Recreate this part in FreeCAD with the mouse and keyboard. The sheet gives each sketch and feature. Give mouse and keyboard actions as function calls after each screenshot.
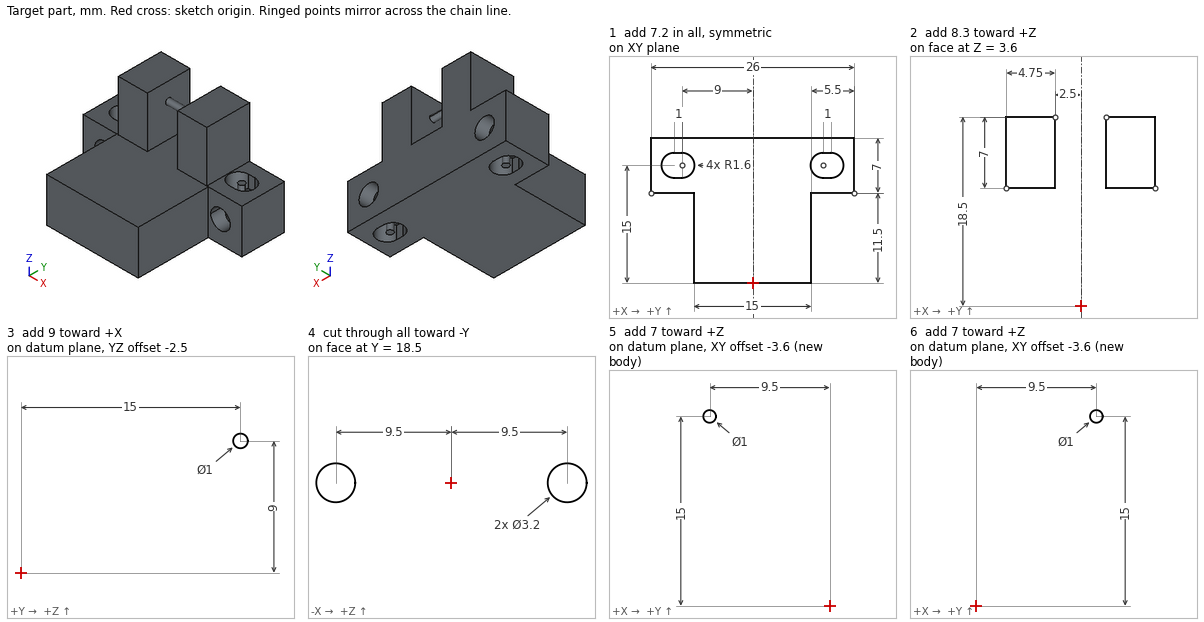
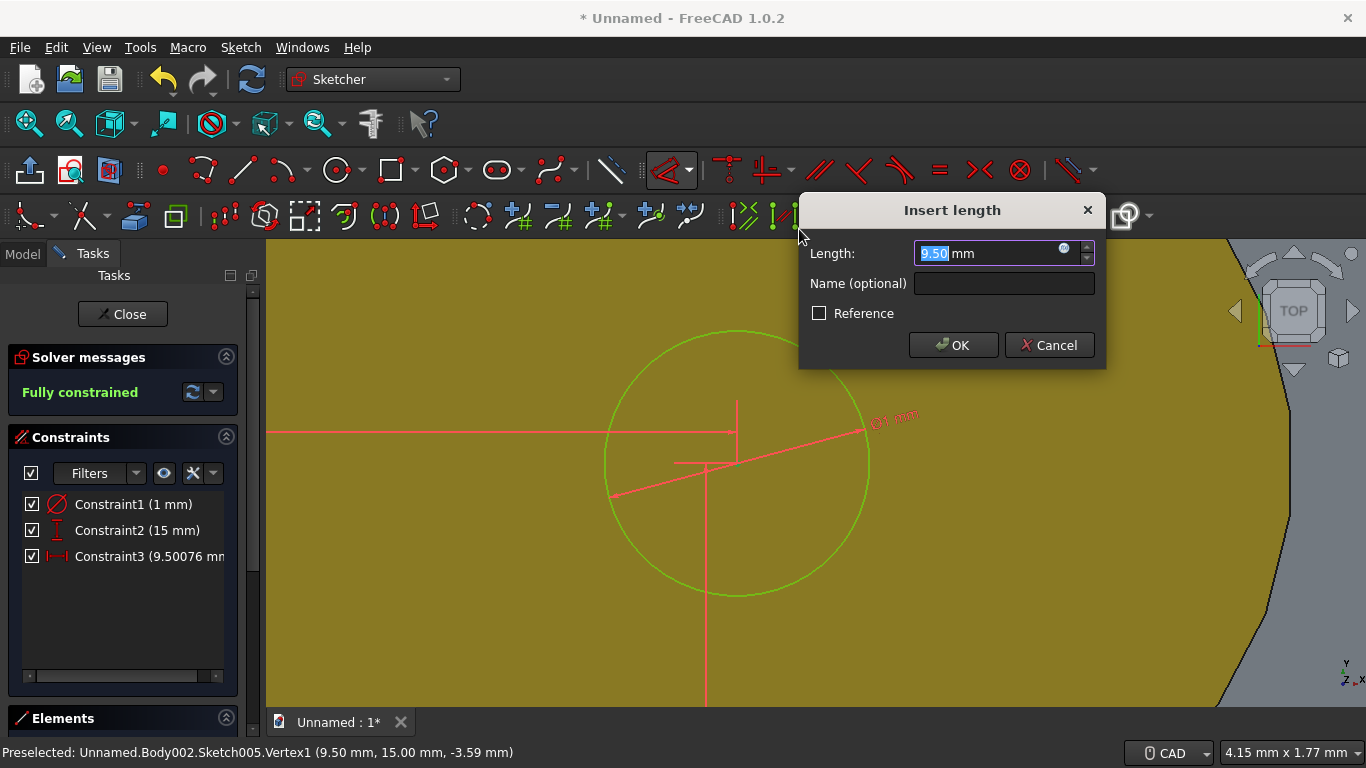
text(9.5)
key(Return)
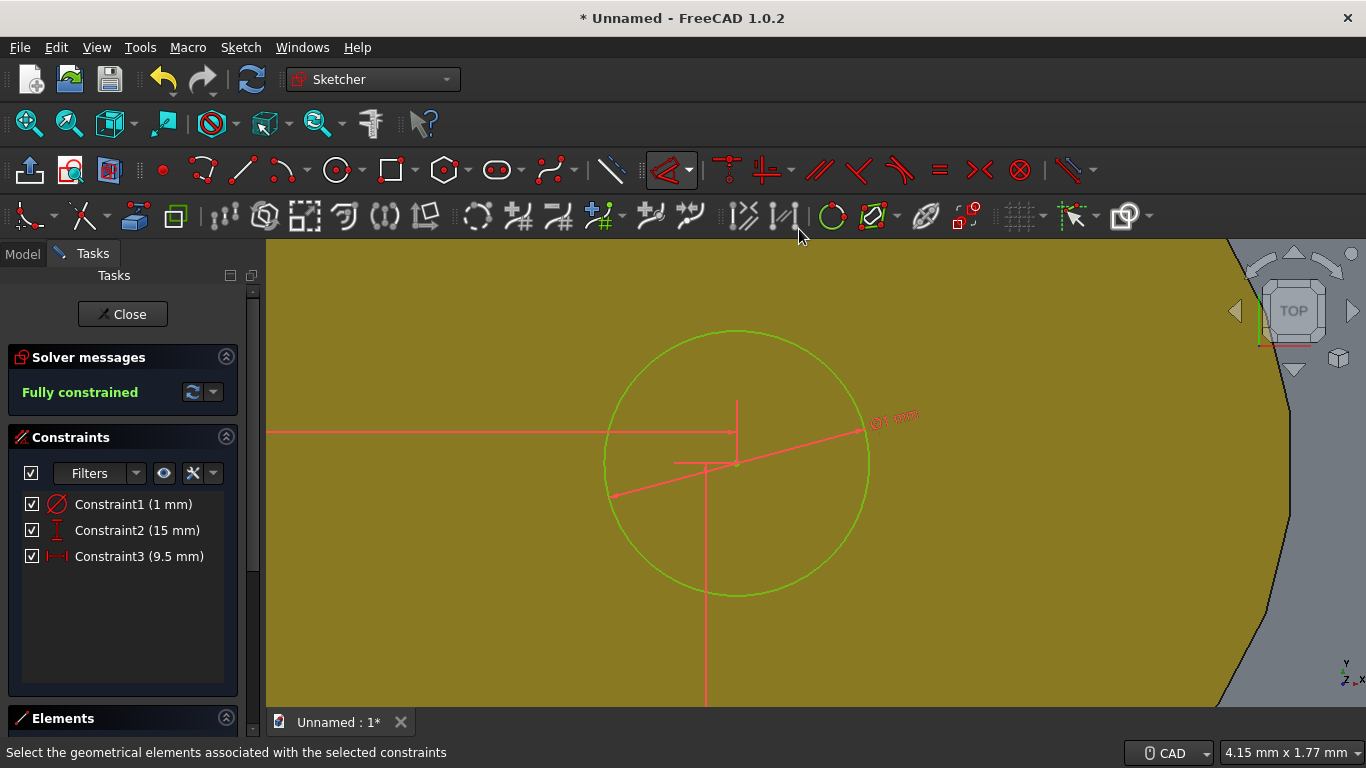
click(123, 314)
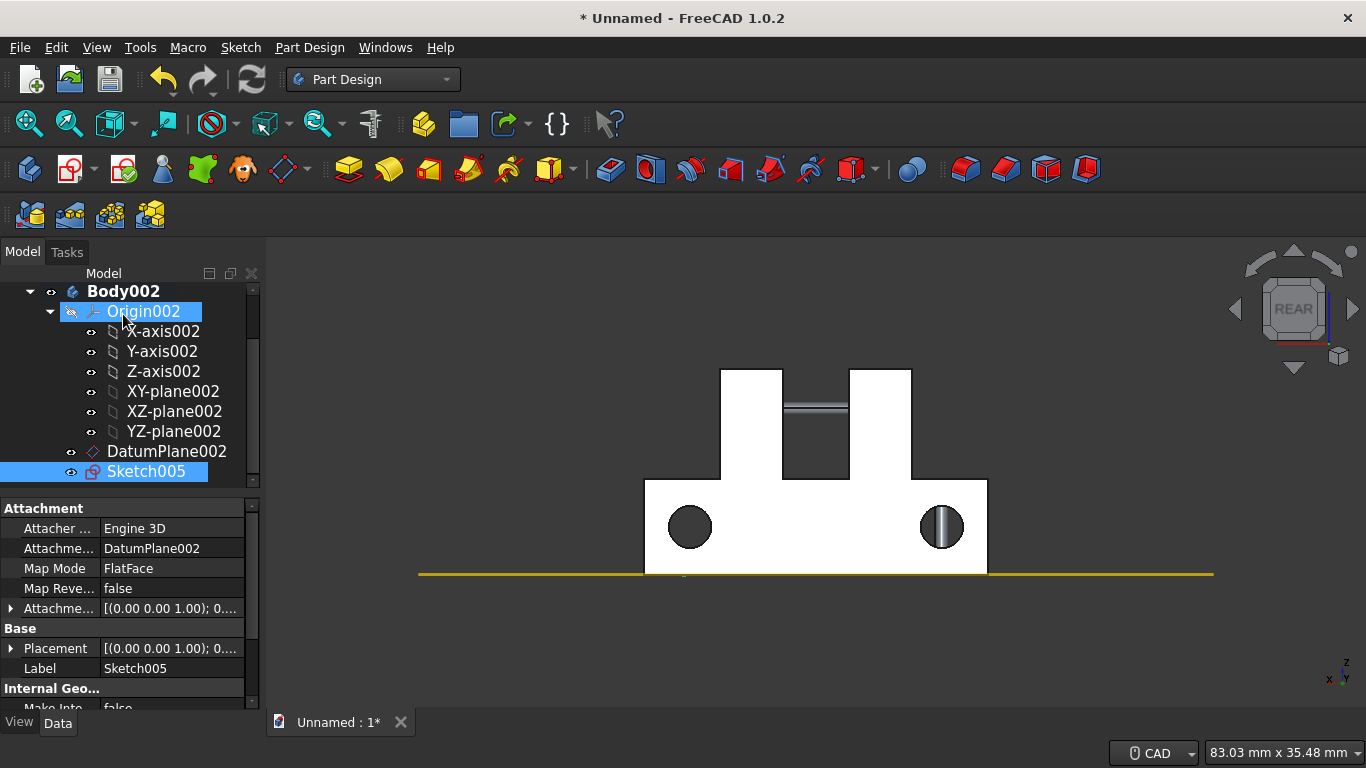
click(350, 170)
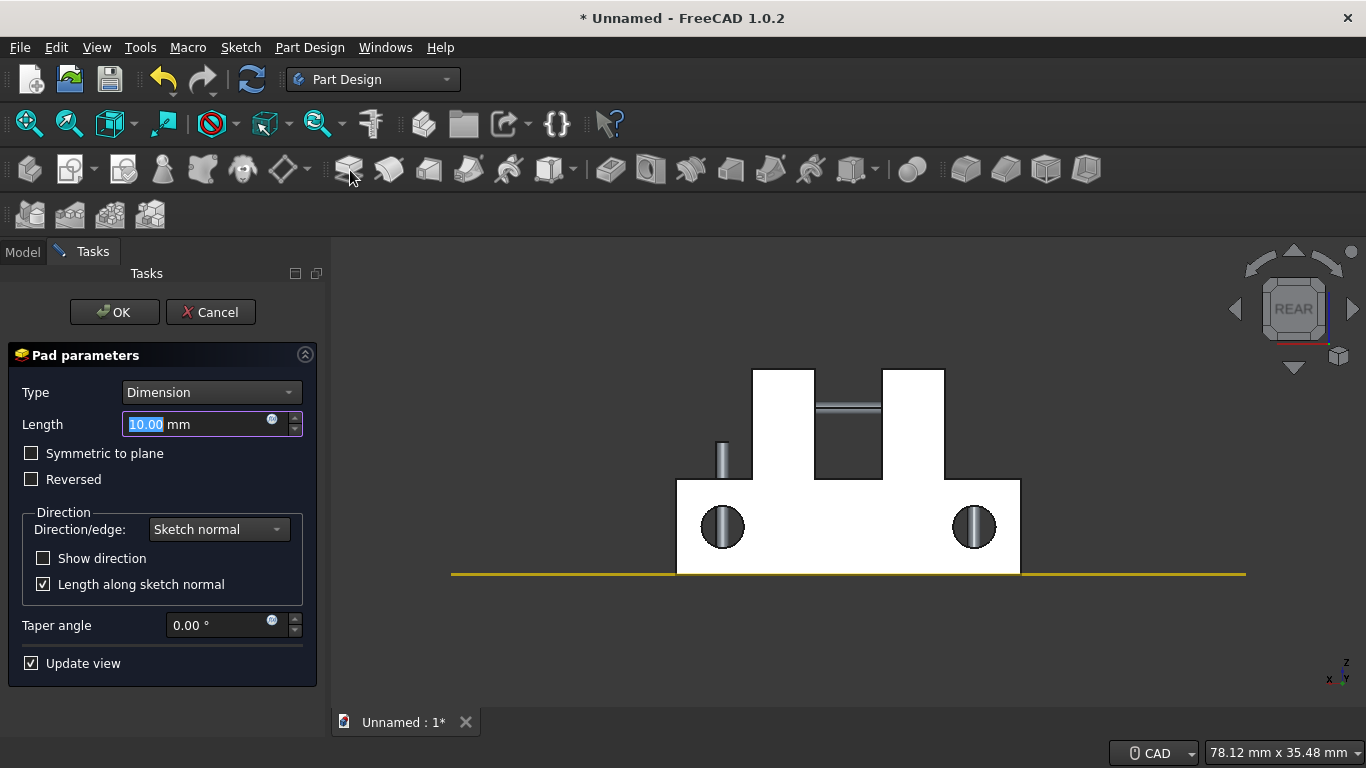
text(7)
key(Tab)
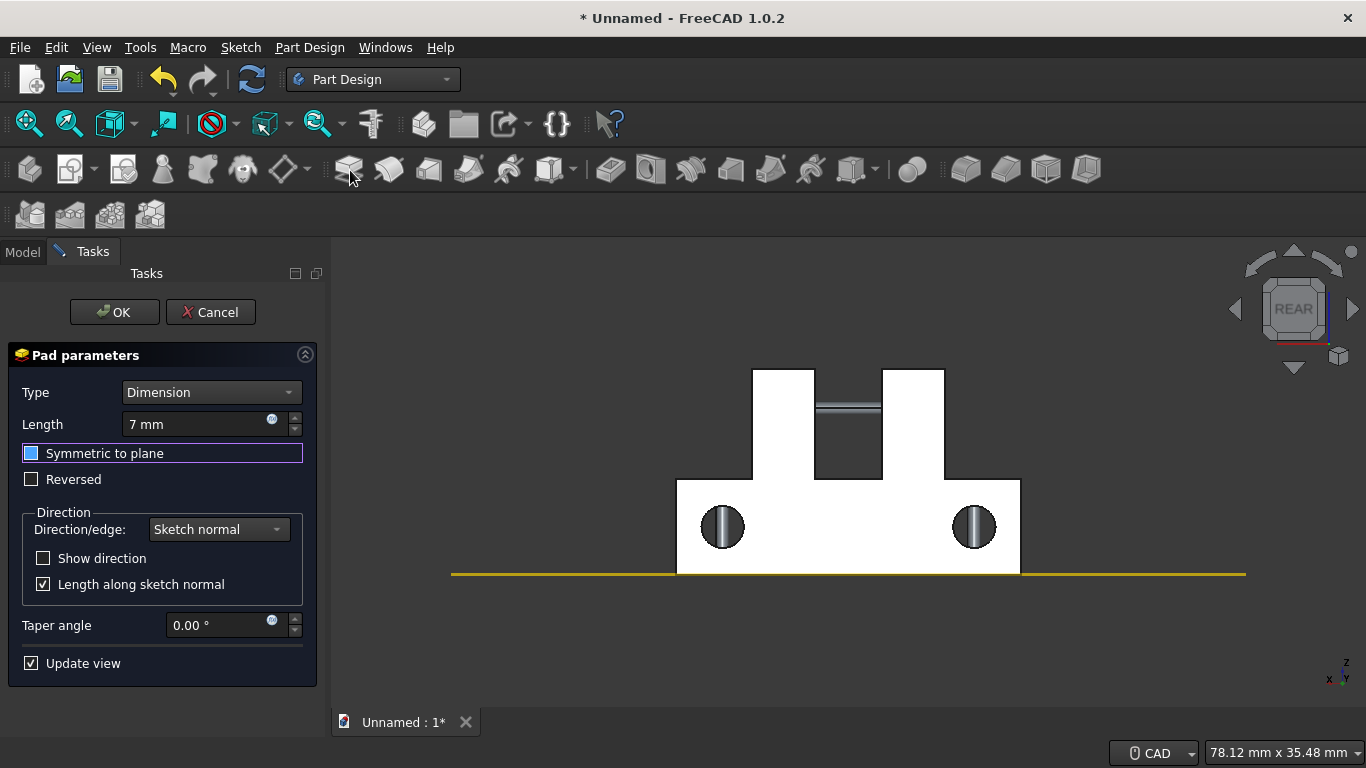
click(115, 312)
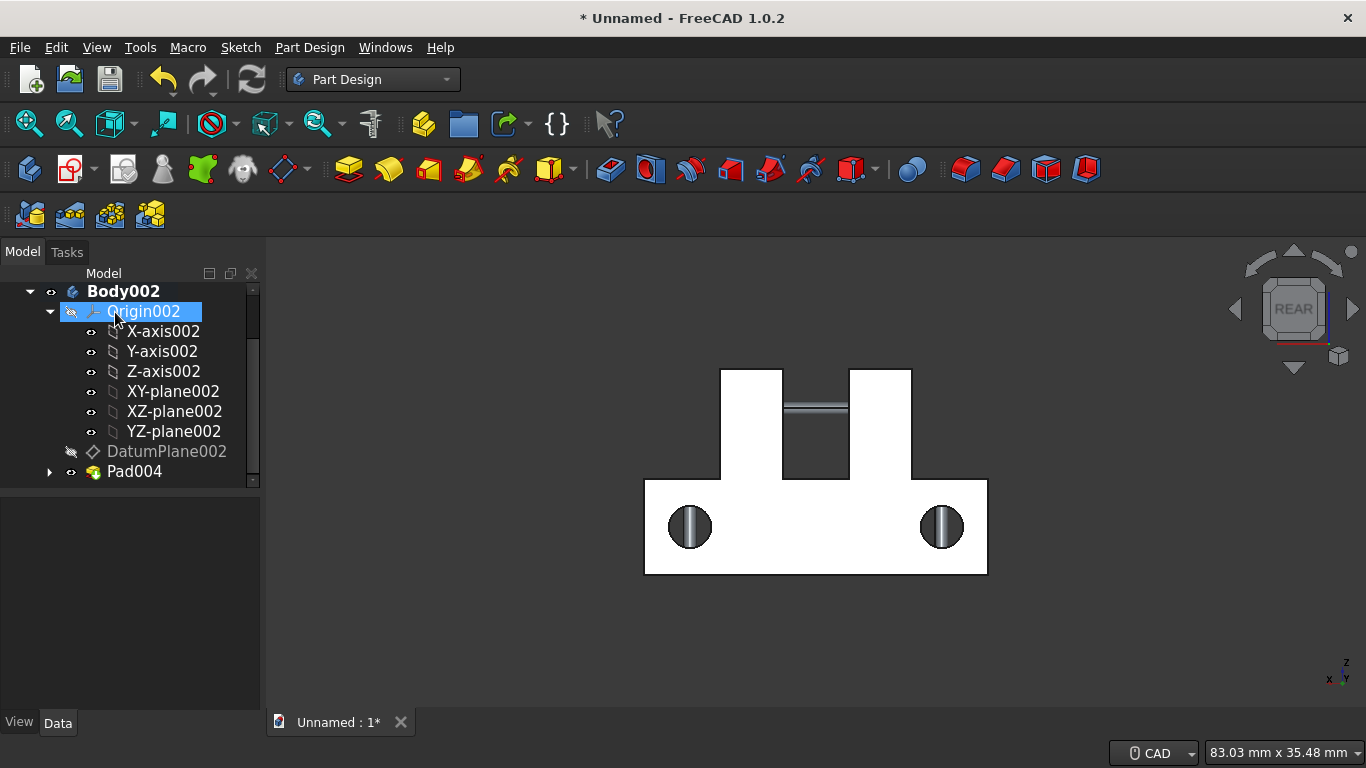
key(0)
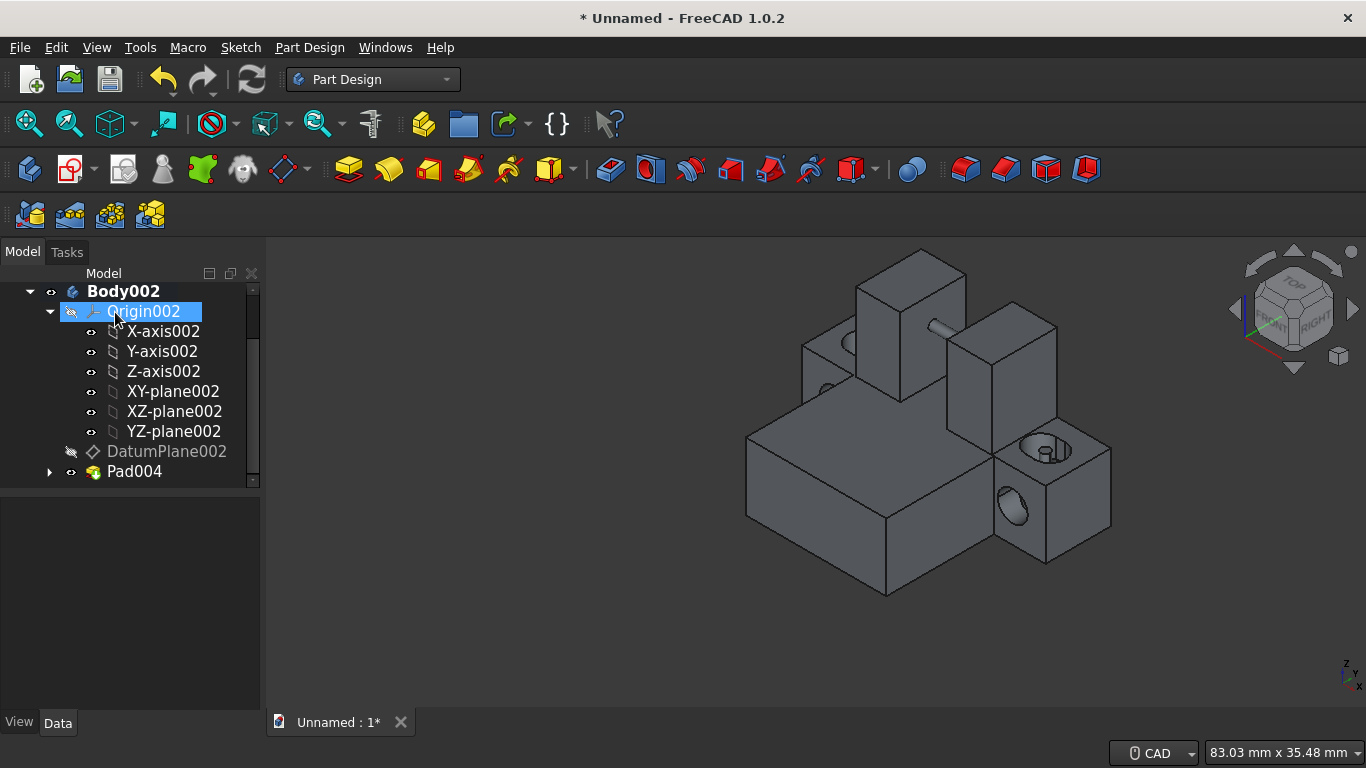
key(v)
key(f)